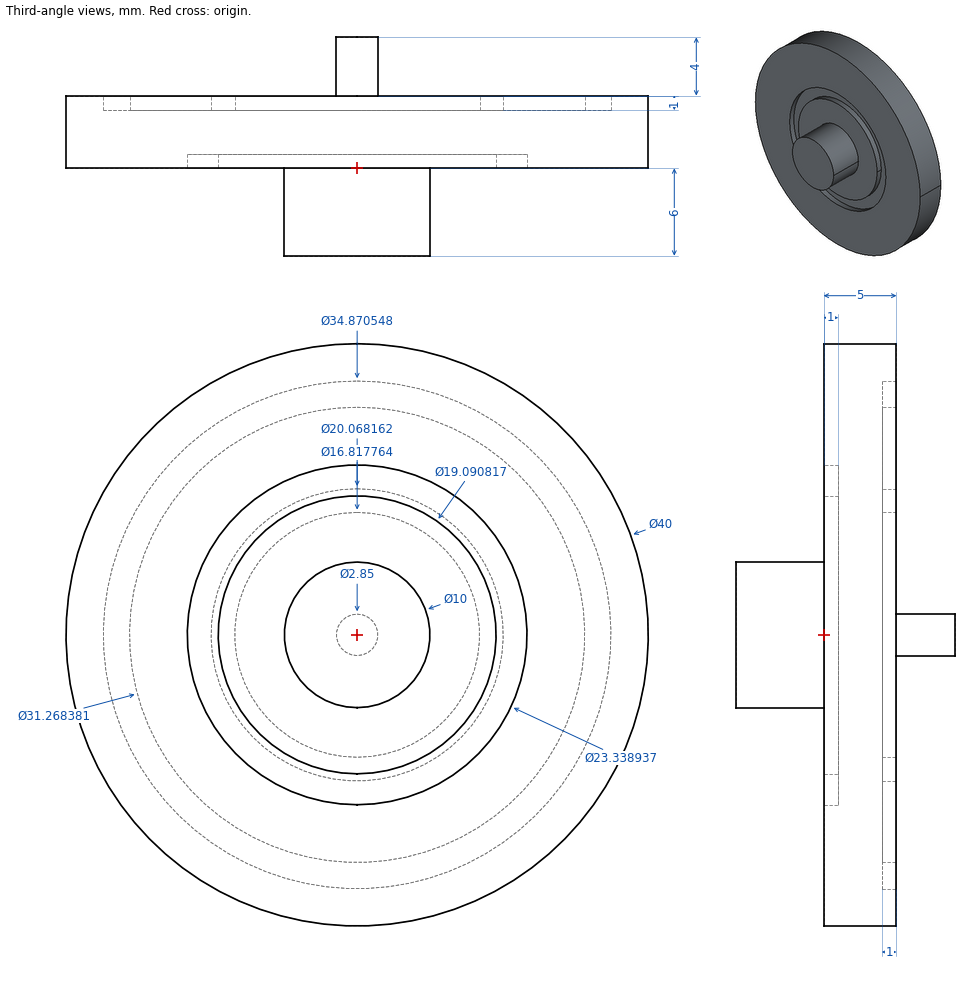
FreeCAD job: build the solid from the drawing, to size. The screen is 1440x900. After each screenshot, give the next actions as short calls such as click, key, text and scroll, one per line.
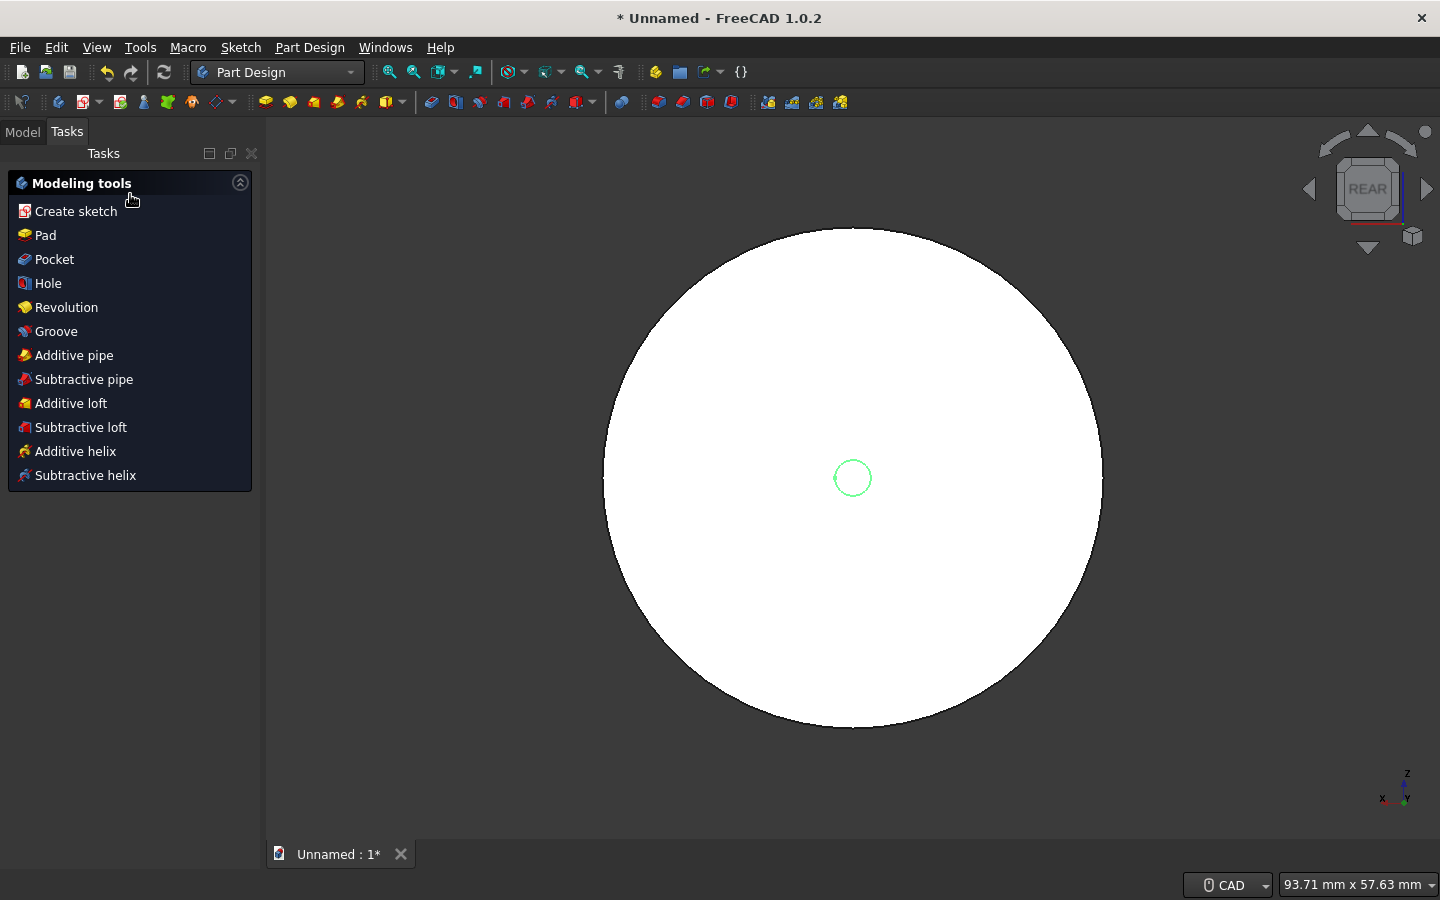
click(266, 102)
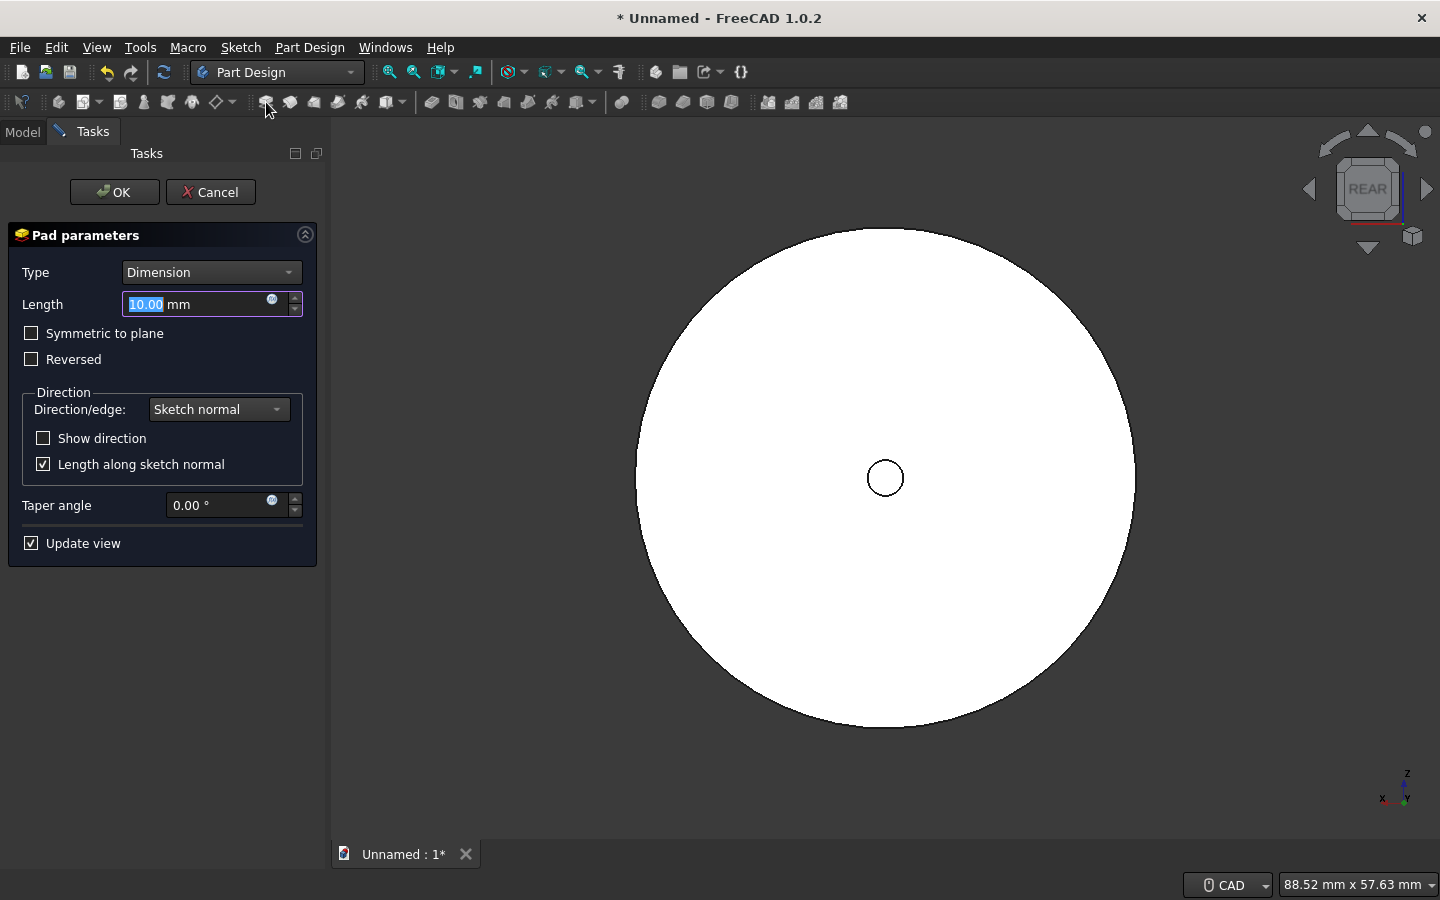
text(4)
key(Tab)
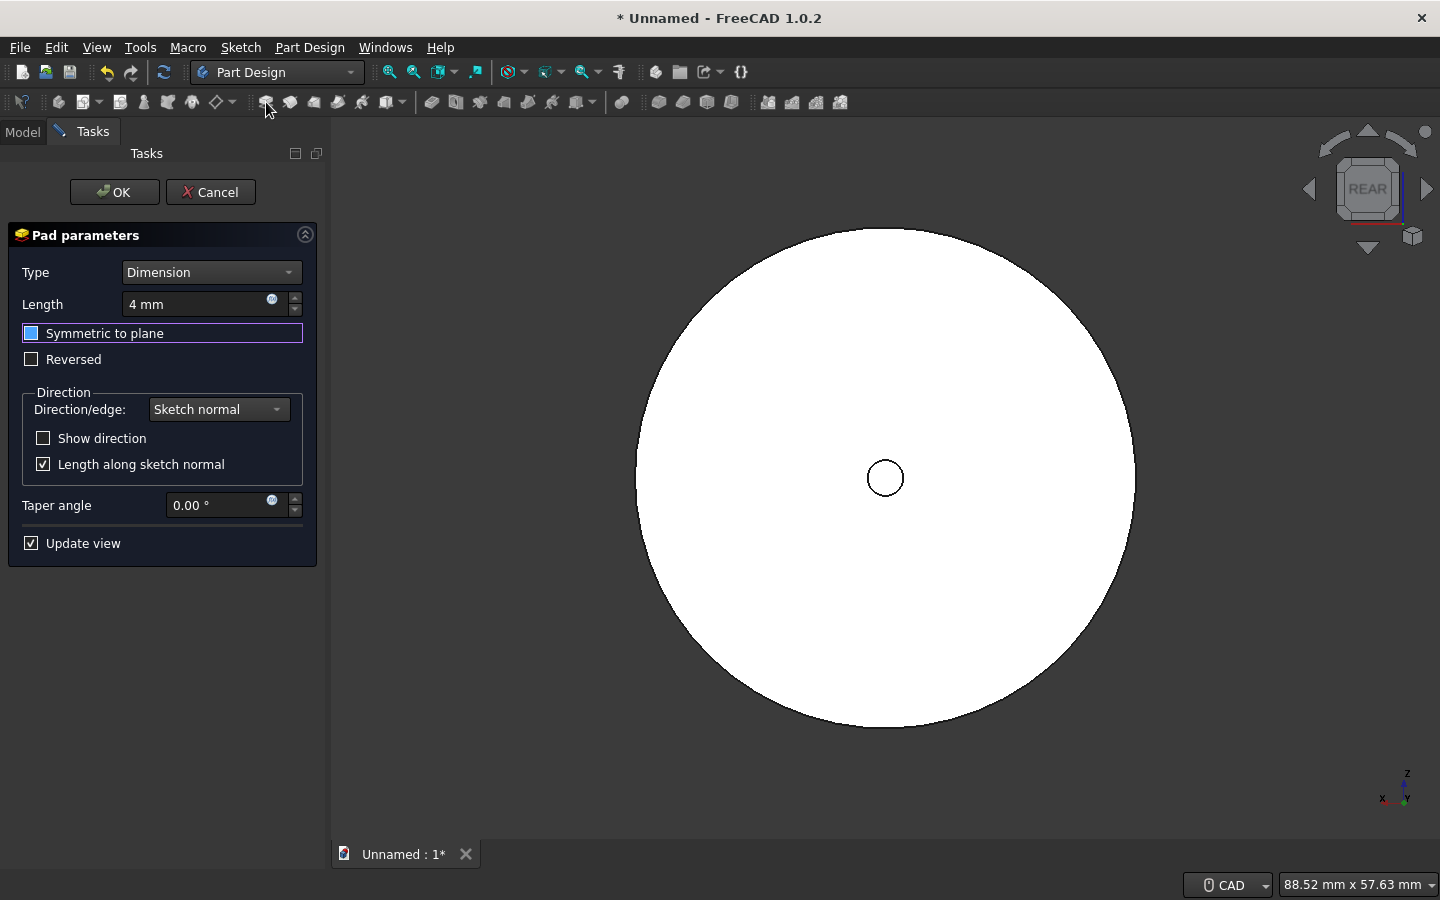
click(115, 192)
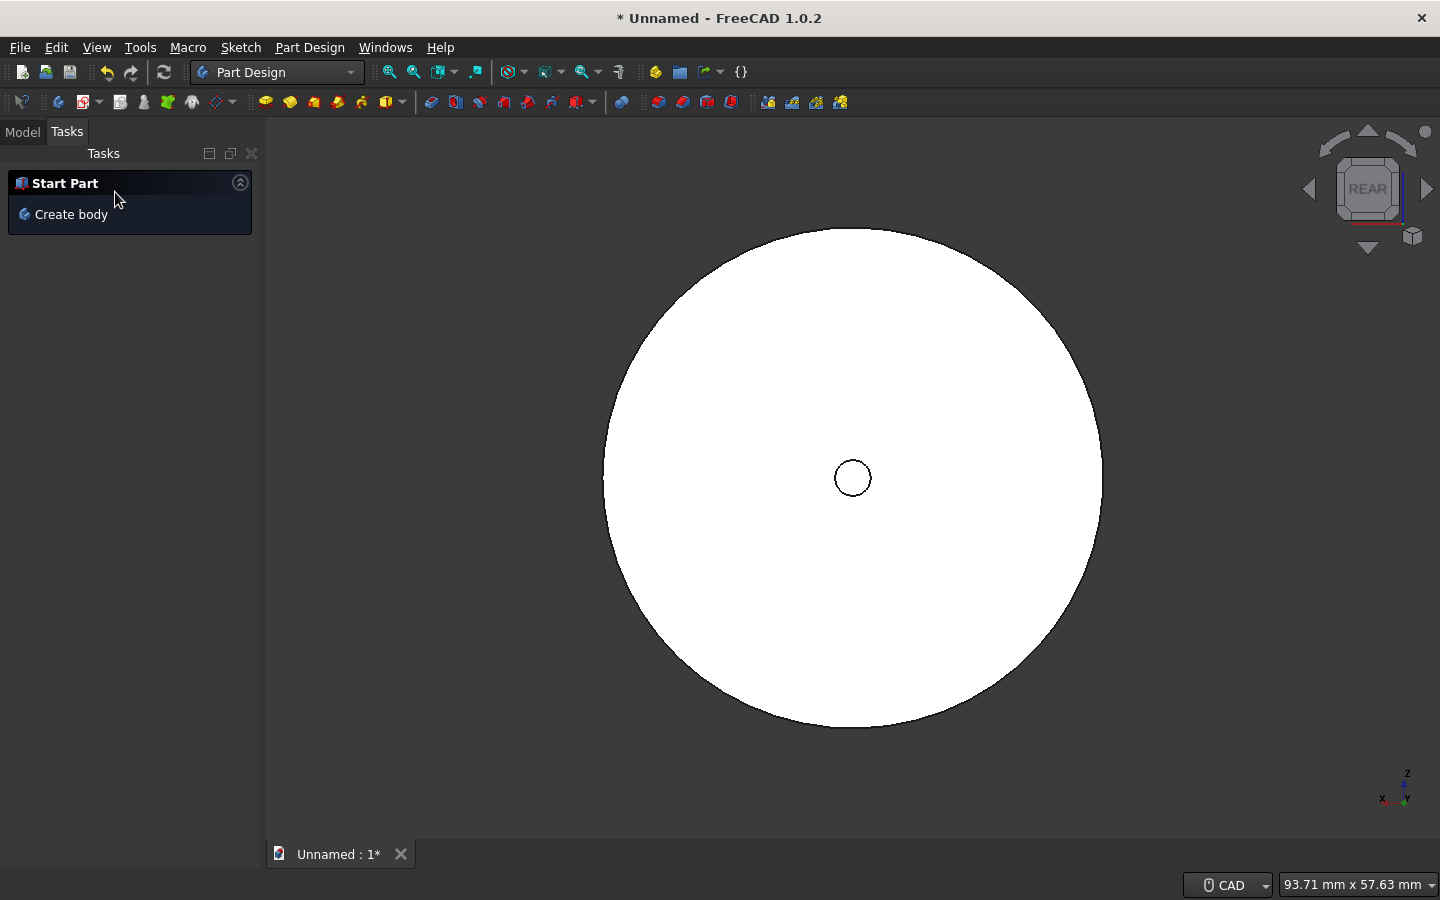
click(710, 477)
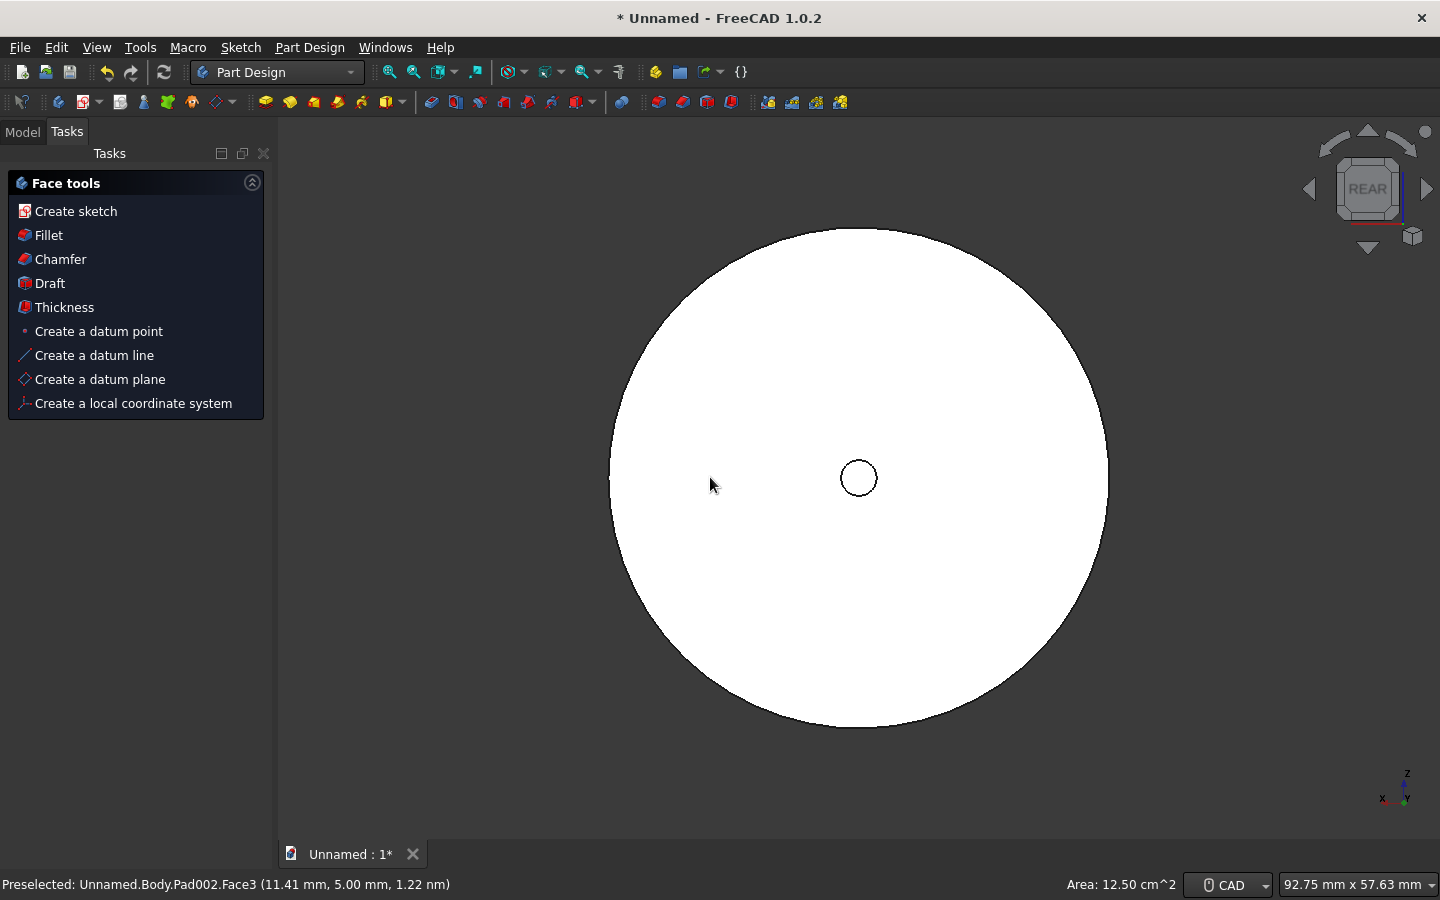
click(84, 102)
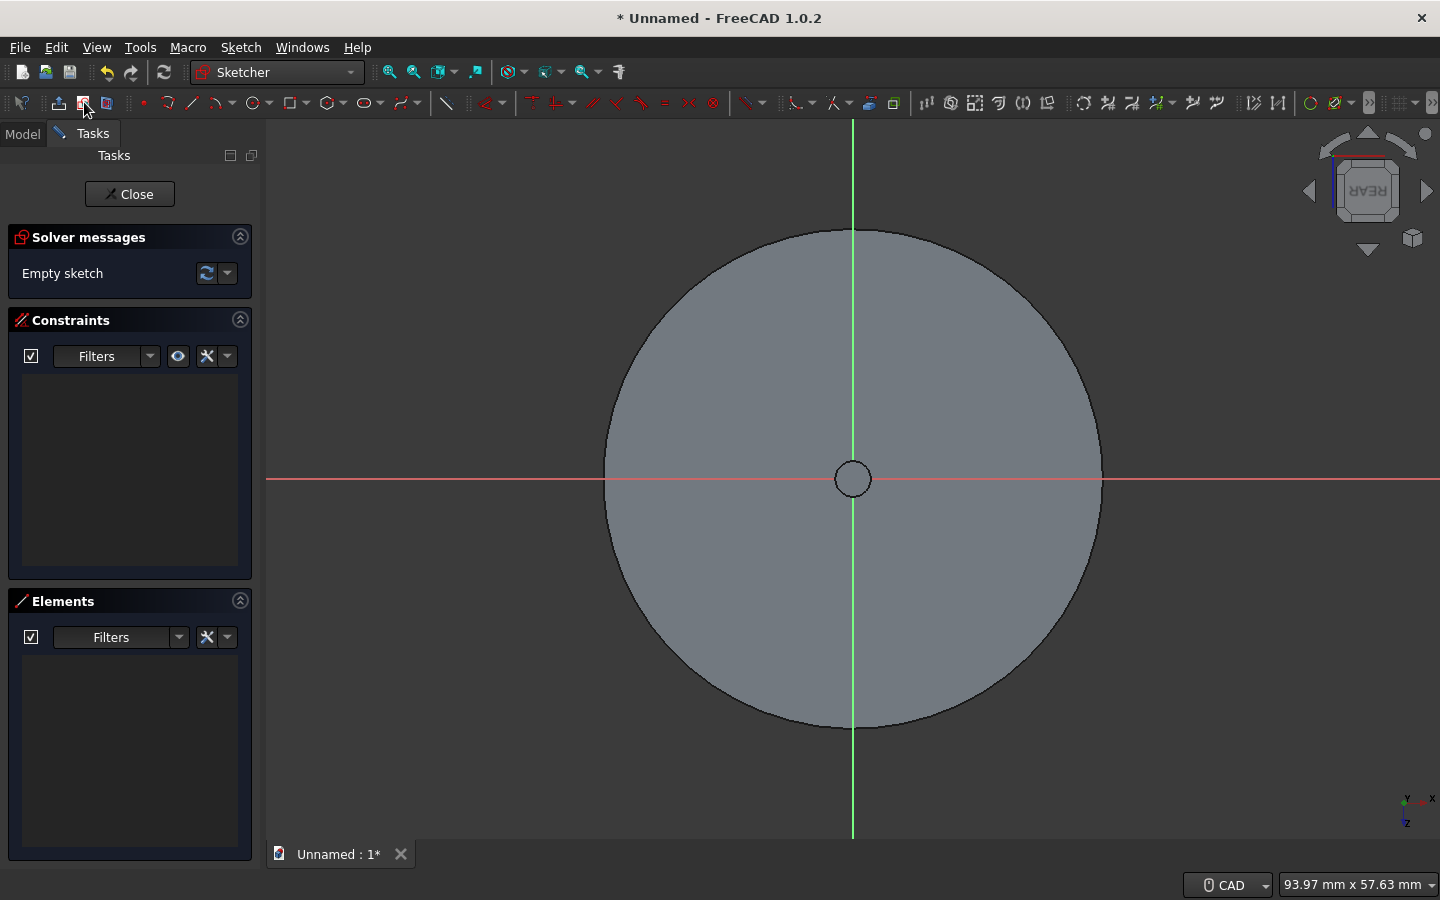
click(108, 104)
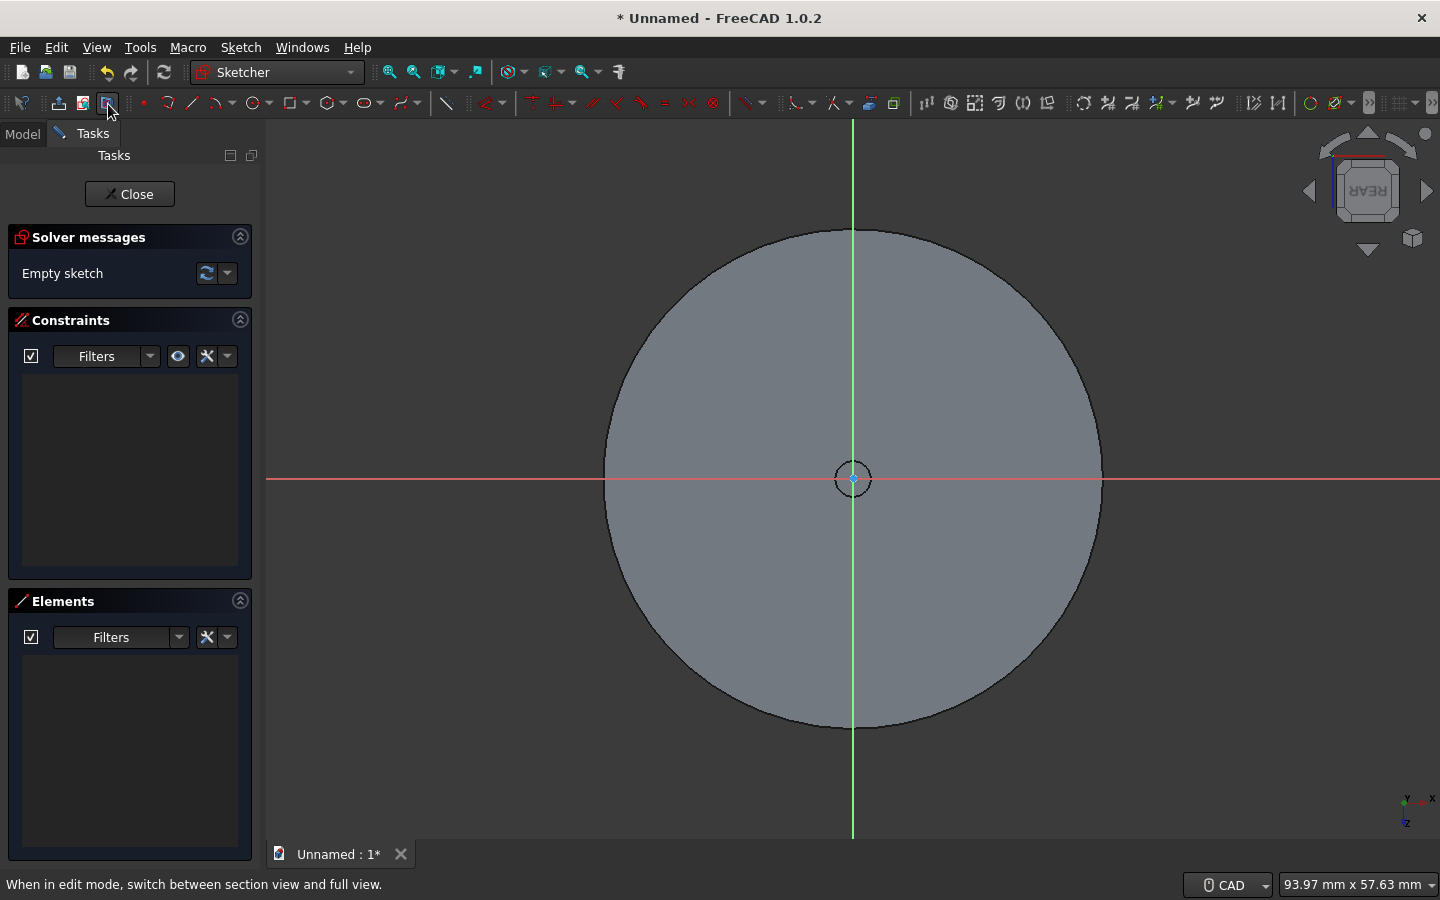
key(g)
key(c)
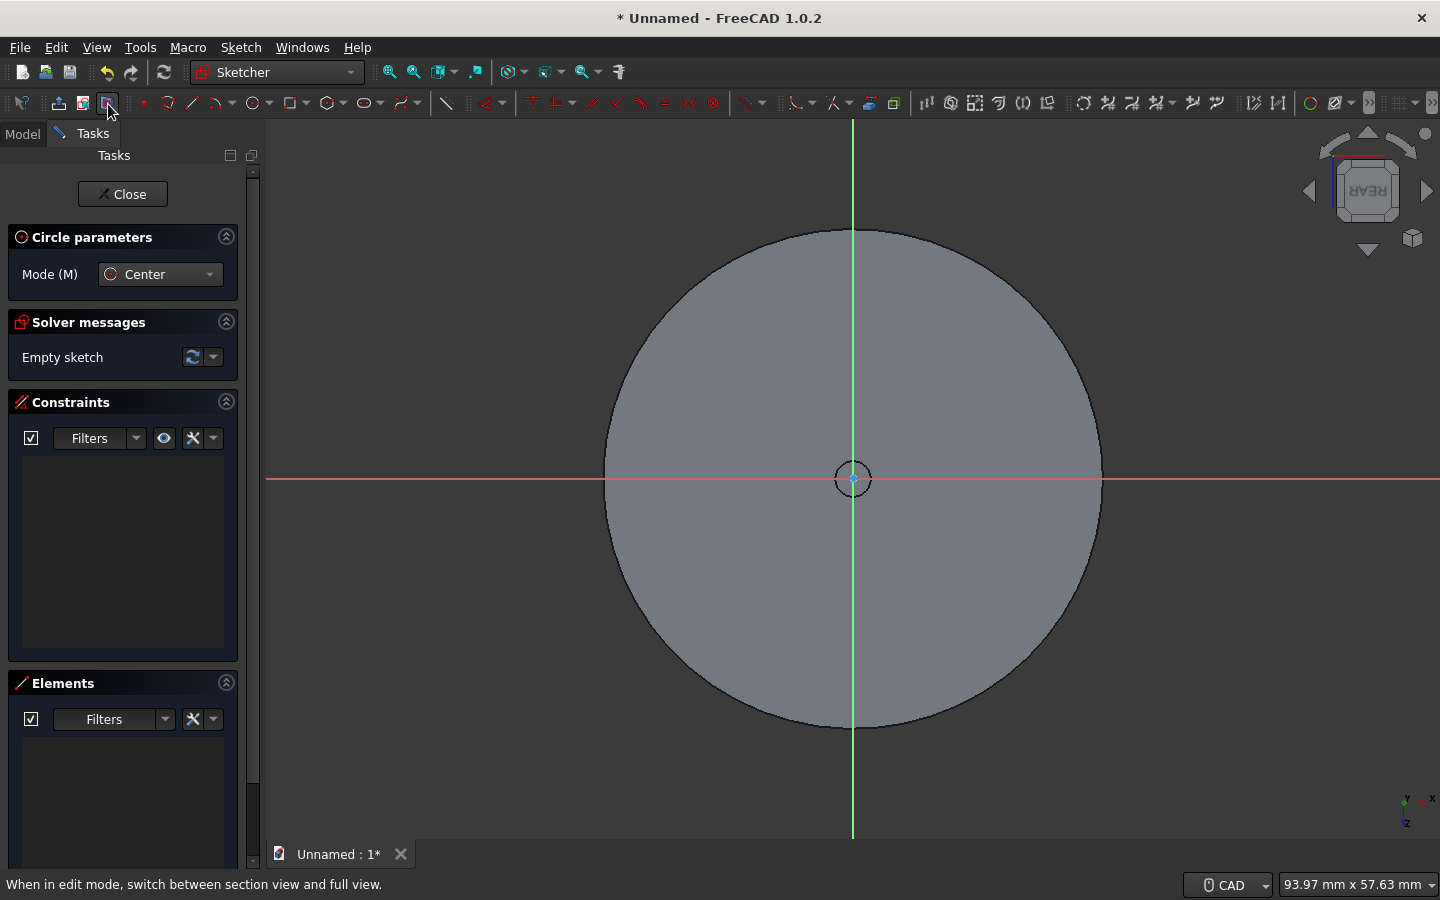
click(853, 479)
click(1007, 325)